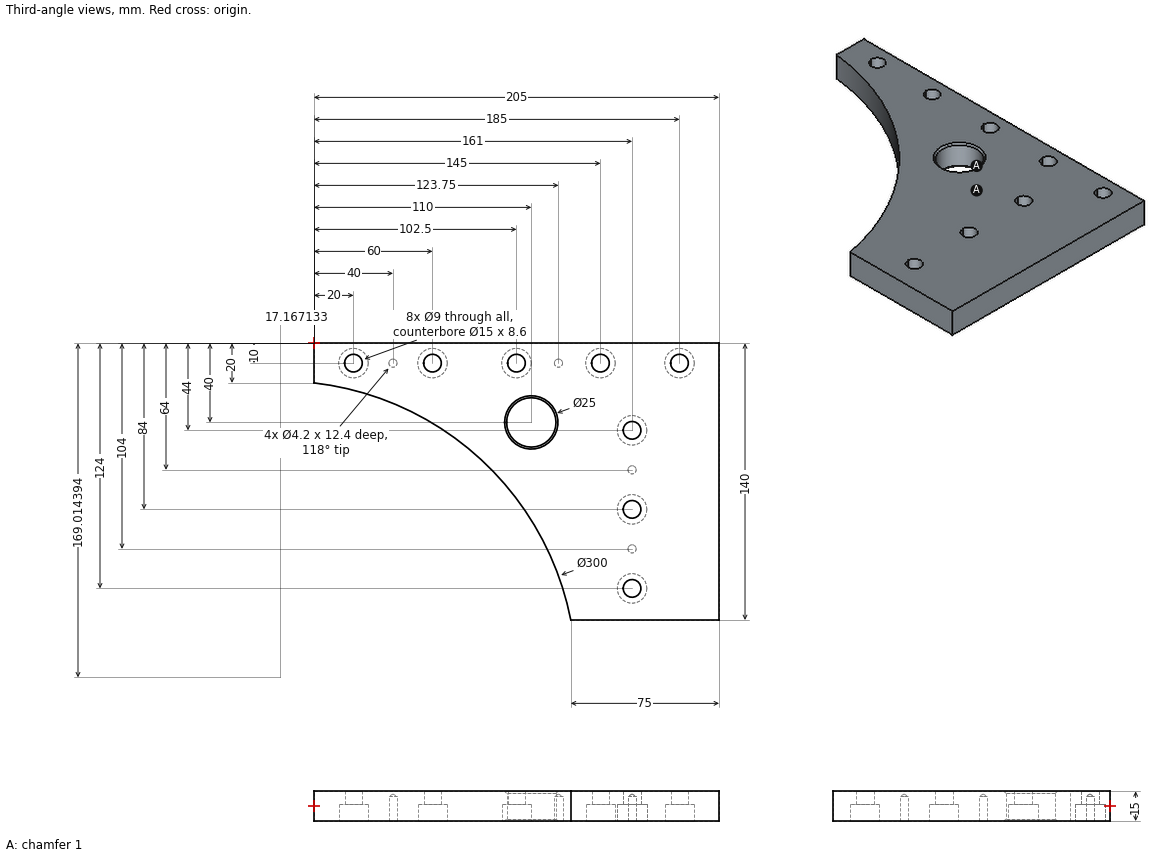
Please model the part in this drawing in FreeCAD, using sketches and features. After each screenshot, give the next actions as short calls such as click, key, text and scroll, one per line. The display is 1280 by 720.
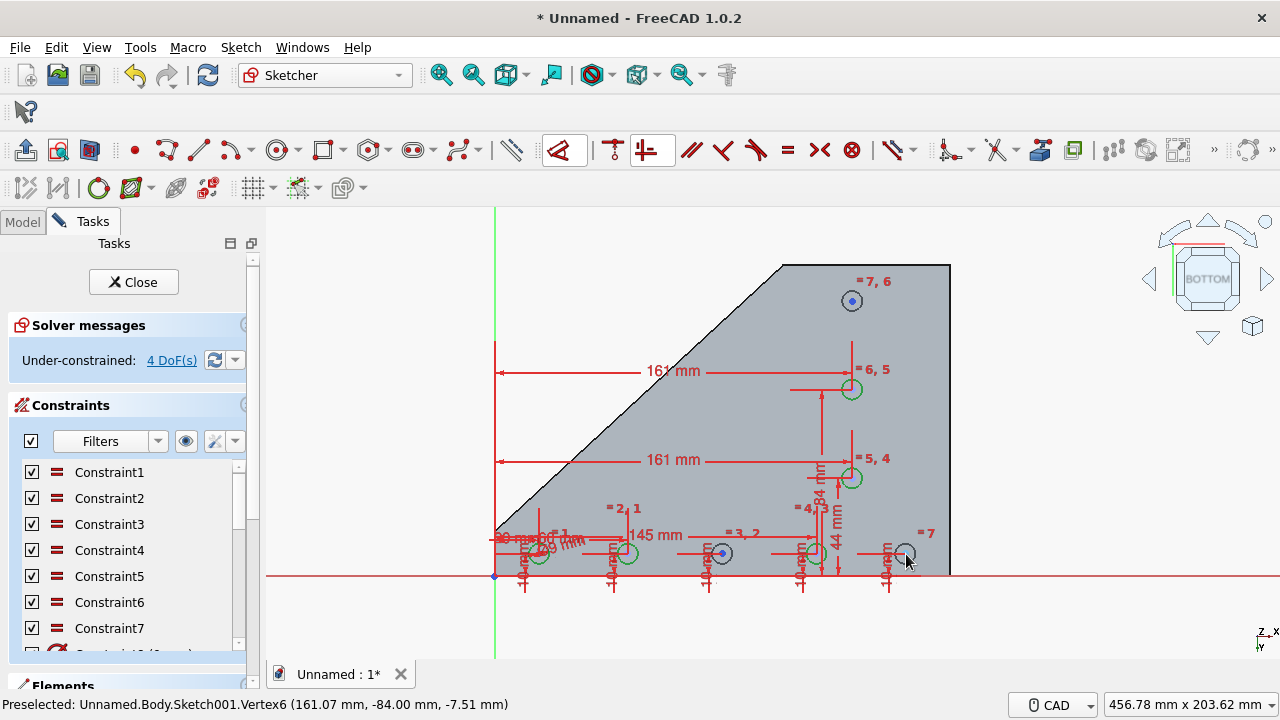
click(852, 301)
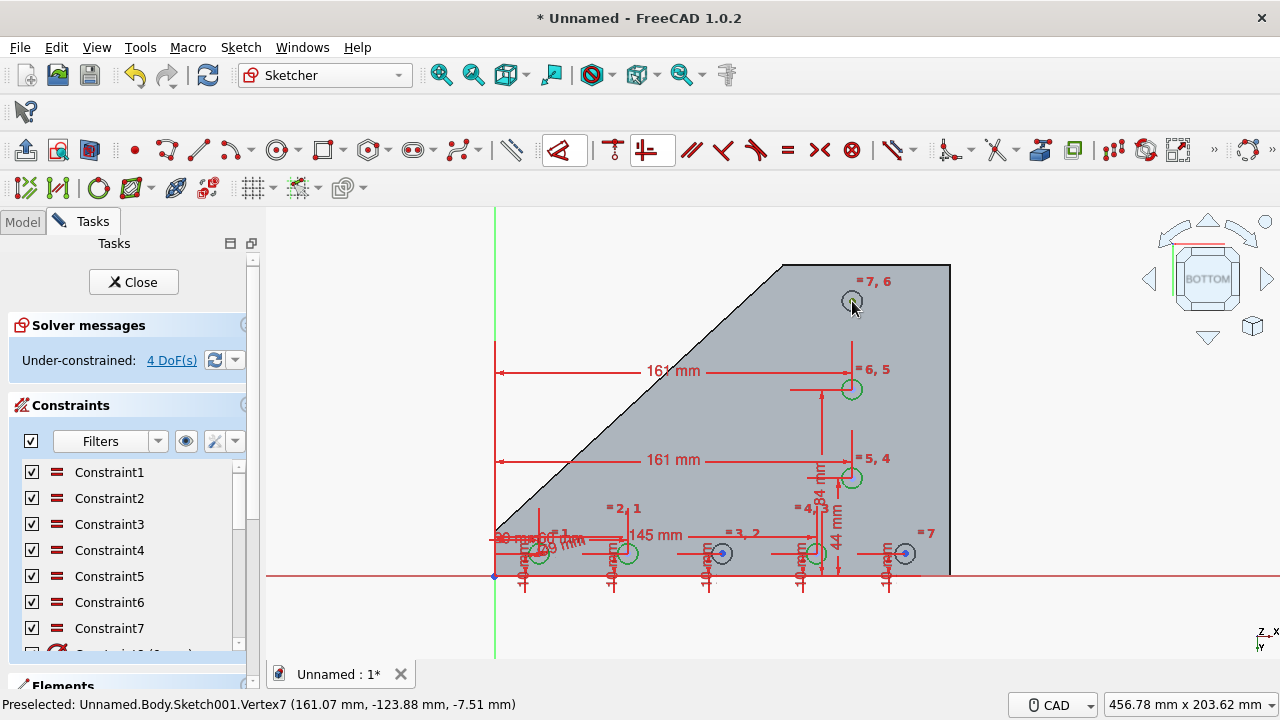
click(582, 150)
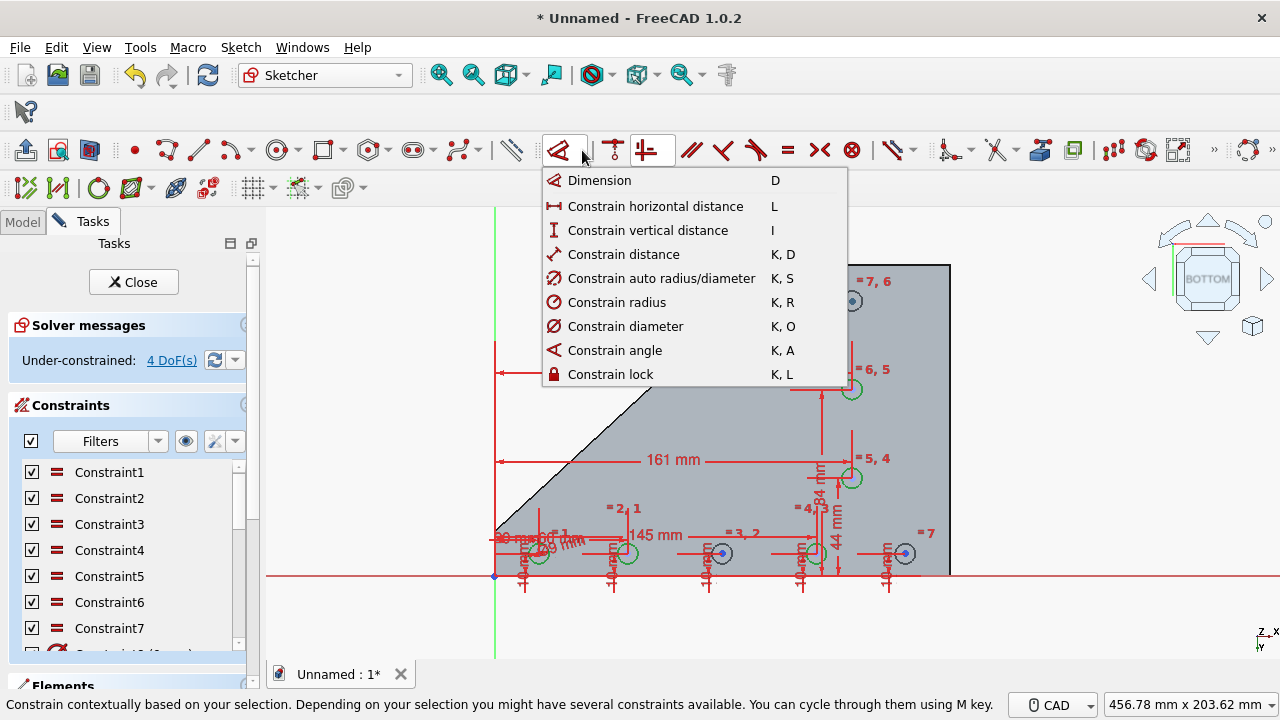
click(695, 206)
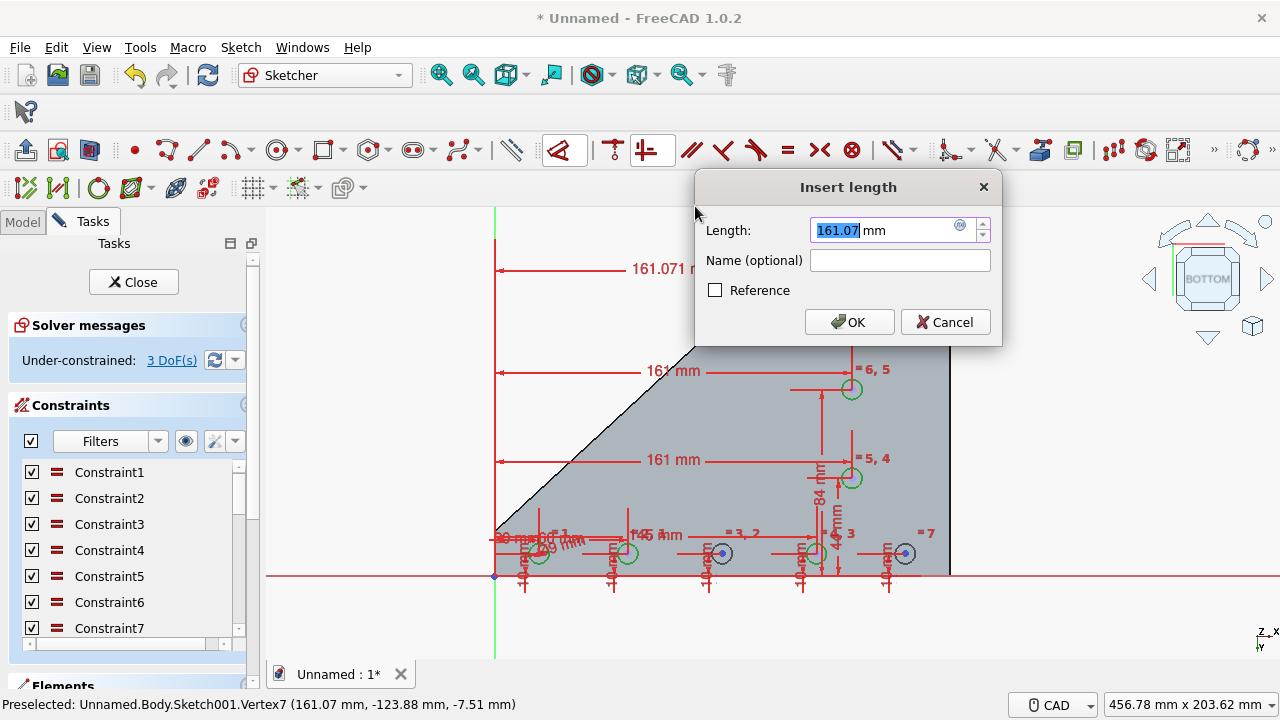
text(161)
key(Return)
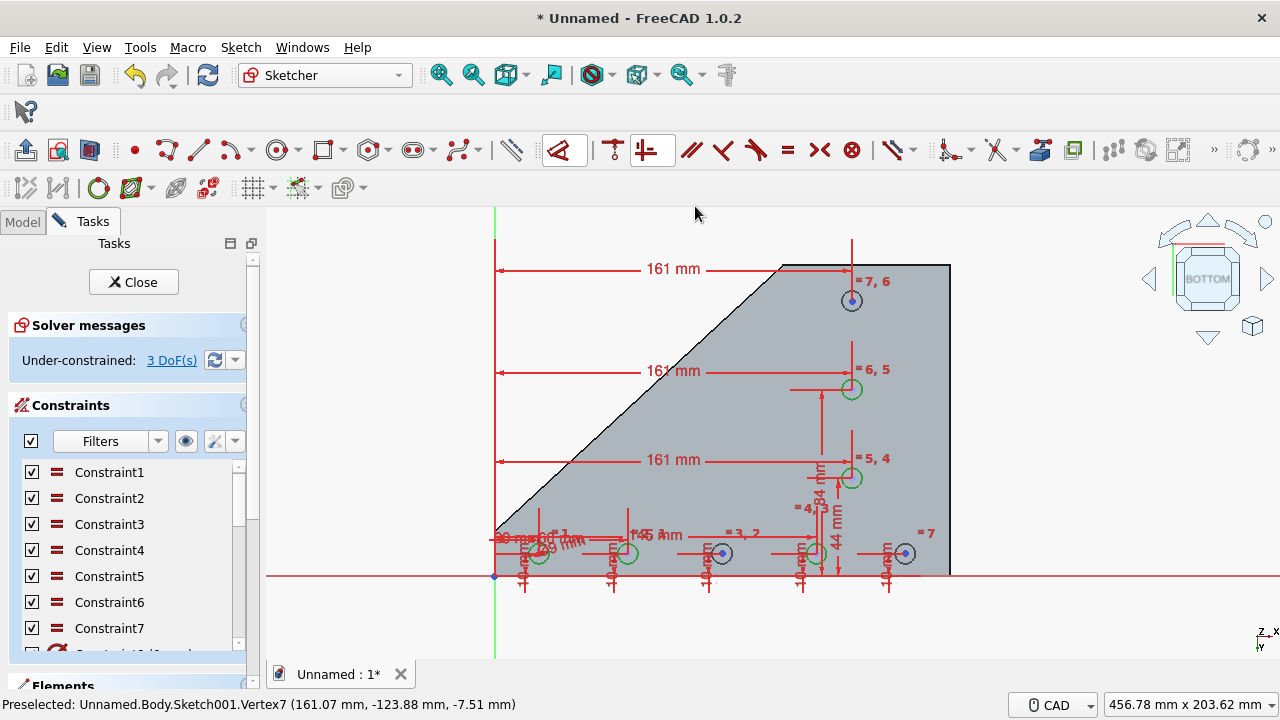
click(852, 301)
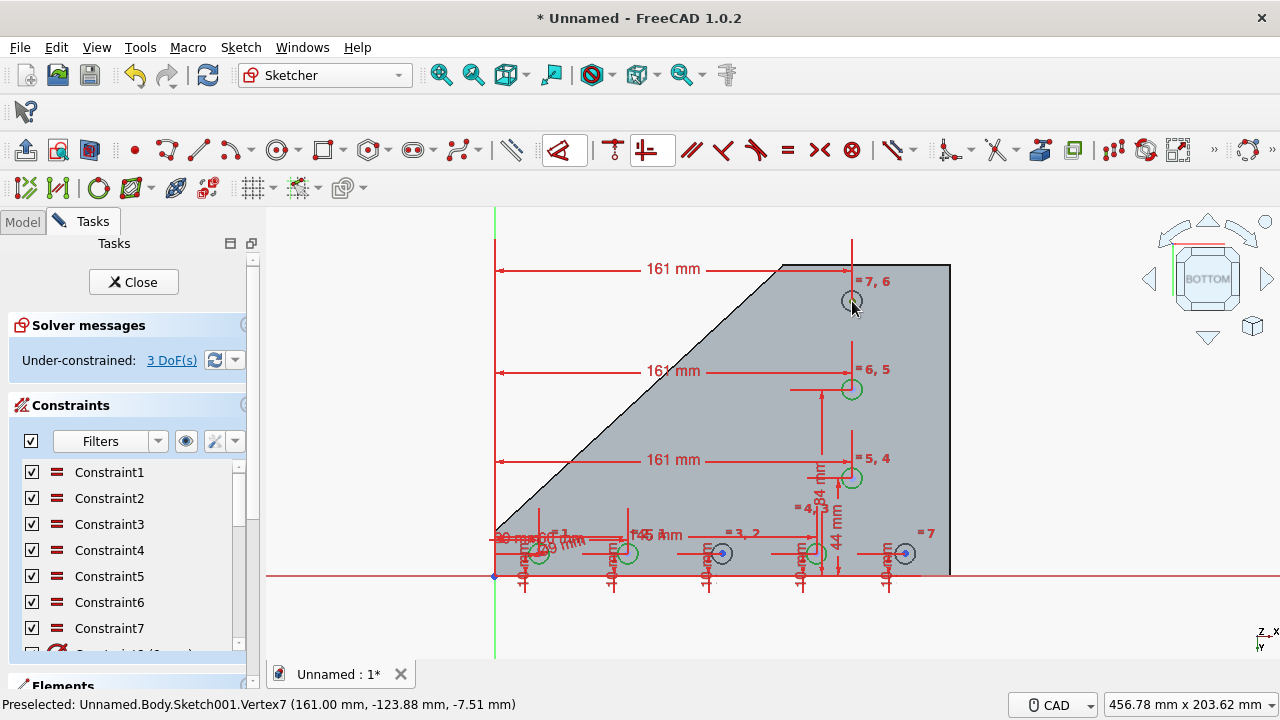
click(582, 150)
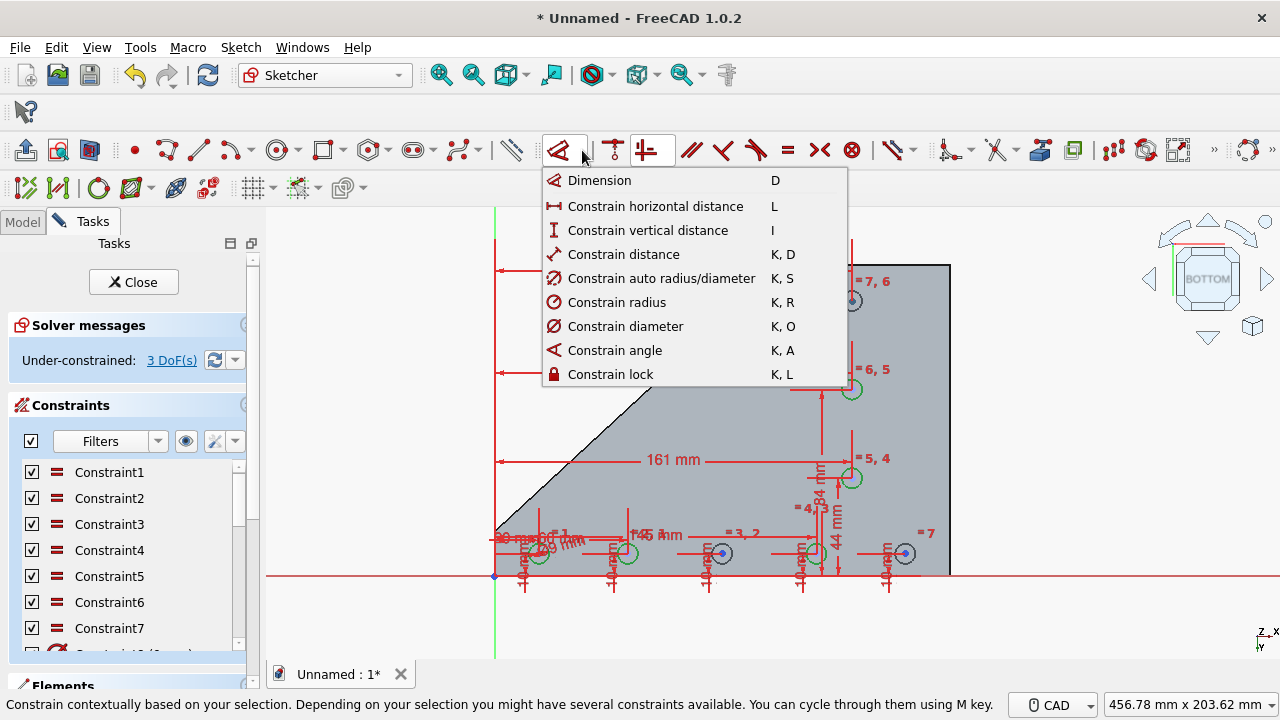
click(695, 230)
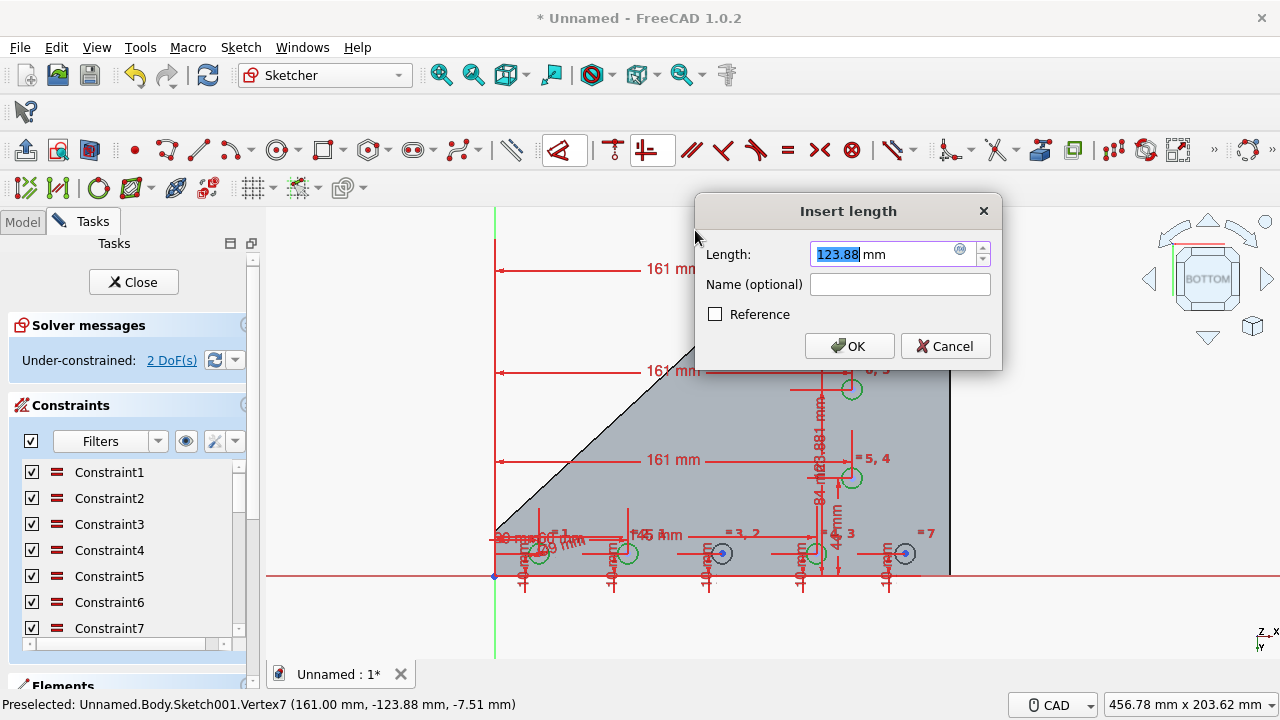
text(124)
key(Return)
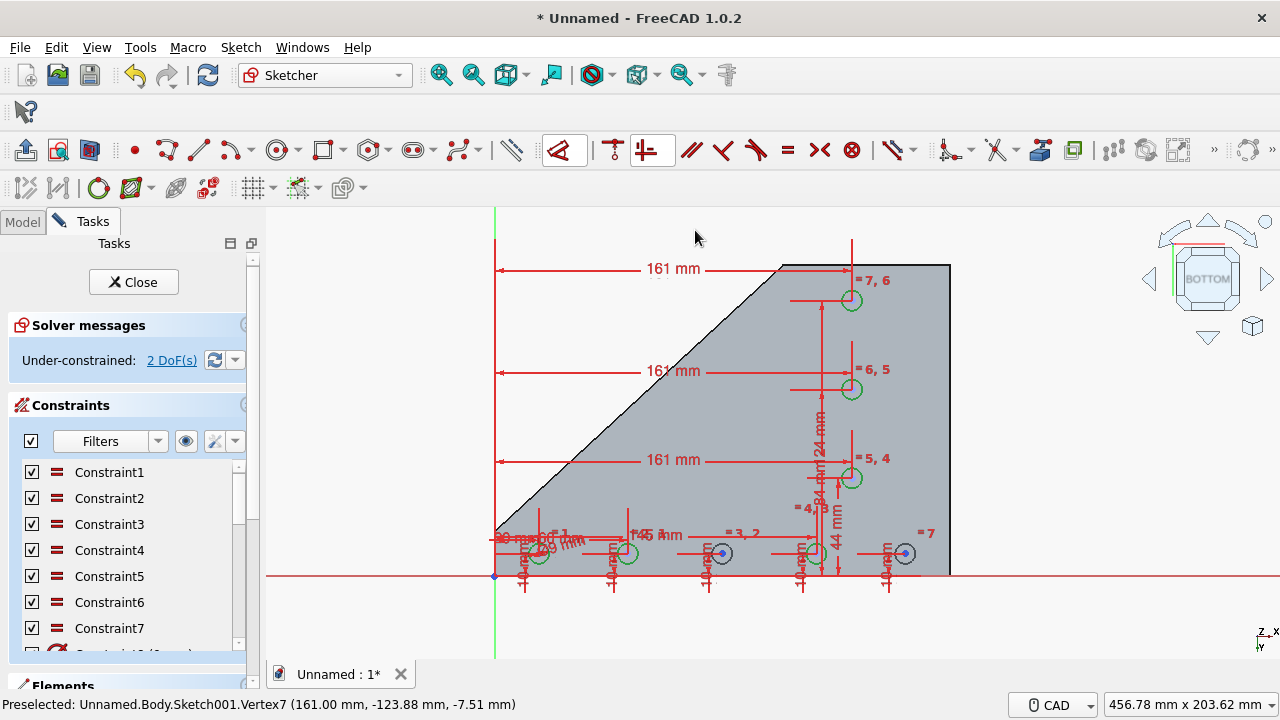
click(905, 554)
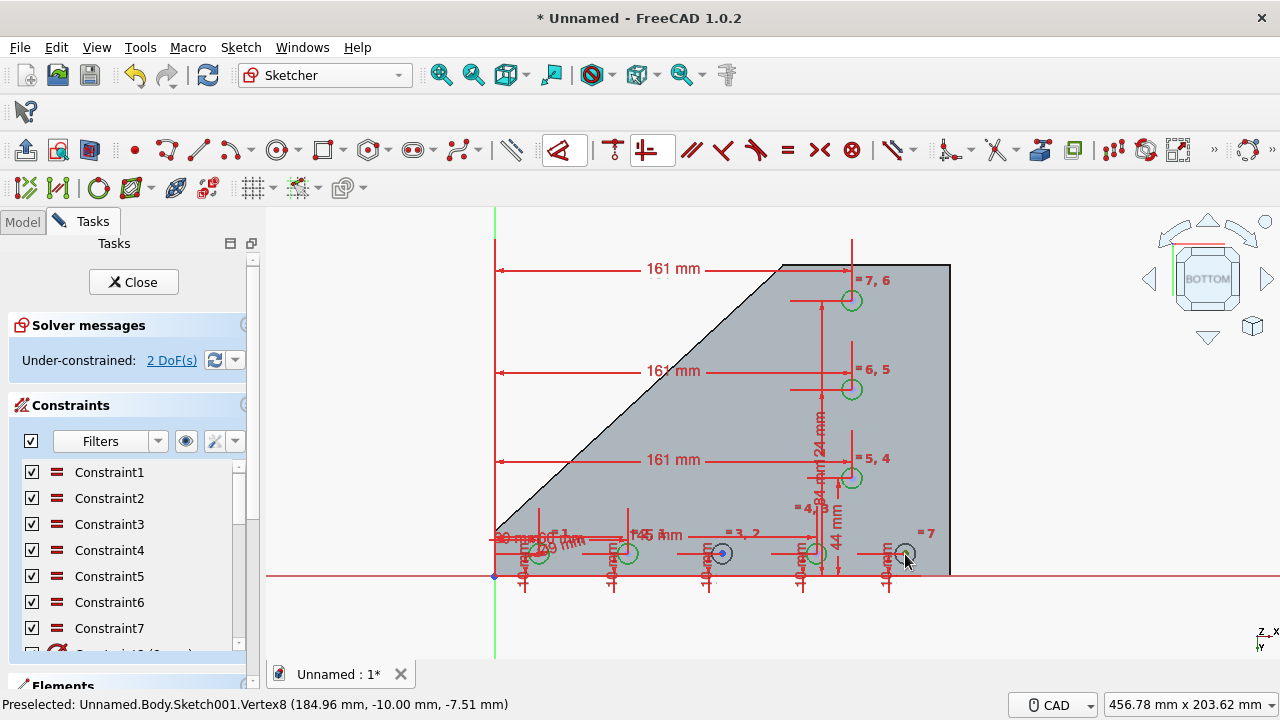
click(582, 150)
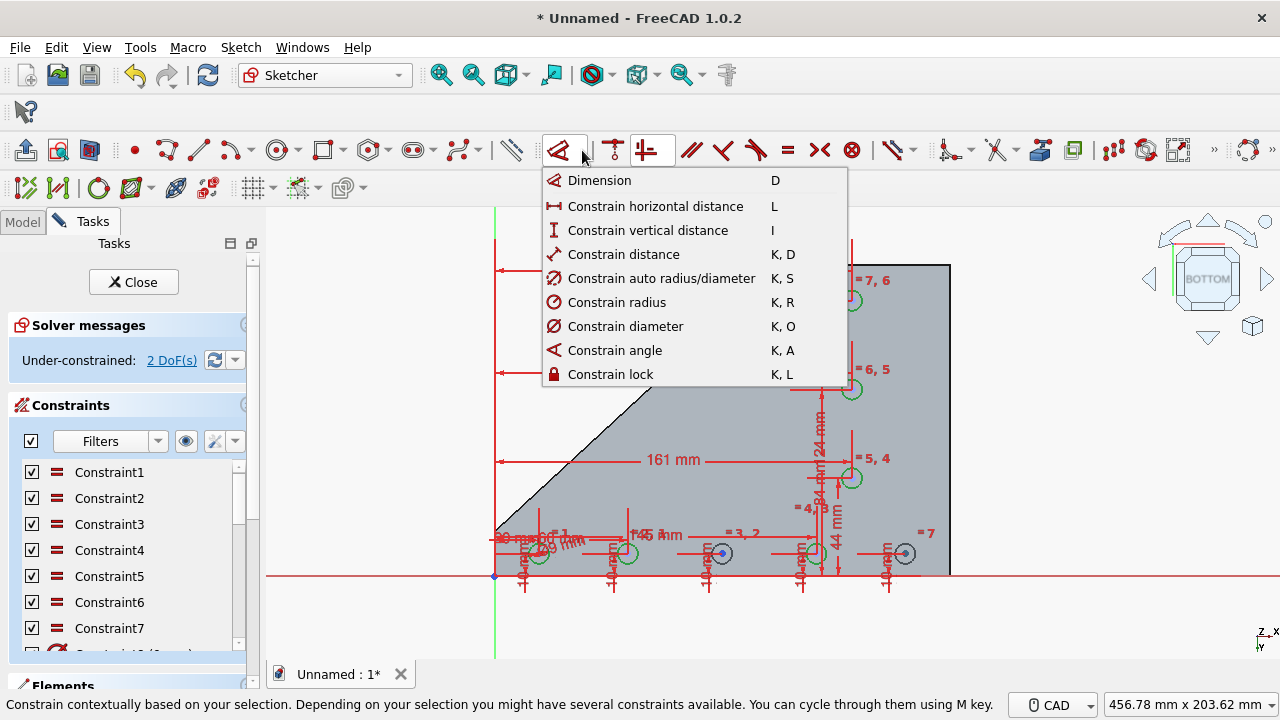
click(695, 206)